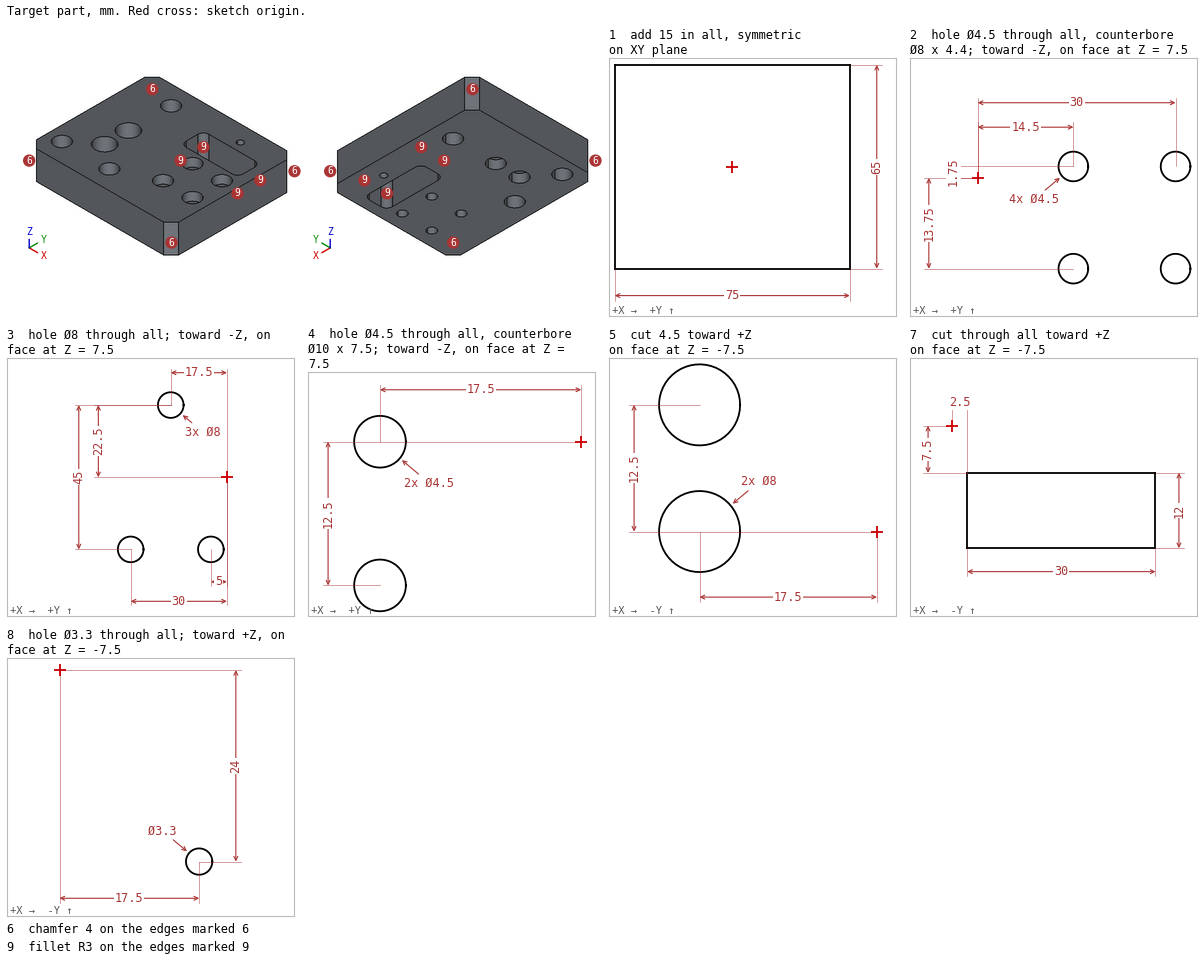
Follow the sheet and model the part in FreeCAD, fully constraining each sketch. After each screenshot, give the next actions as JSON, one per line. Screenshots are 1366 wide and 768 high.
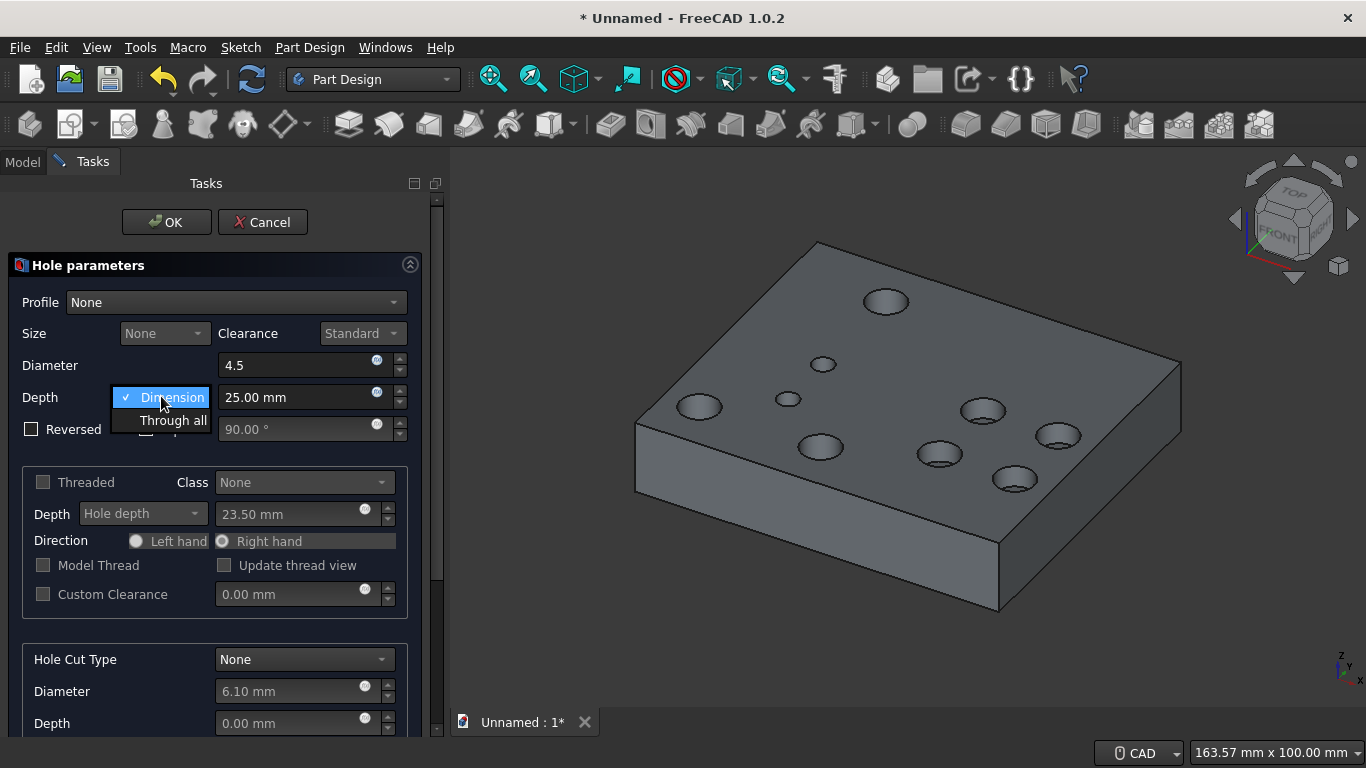
{"action": "left_click", "coordinate": [160, 420]}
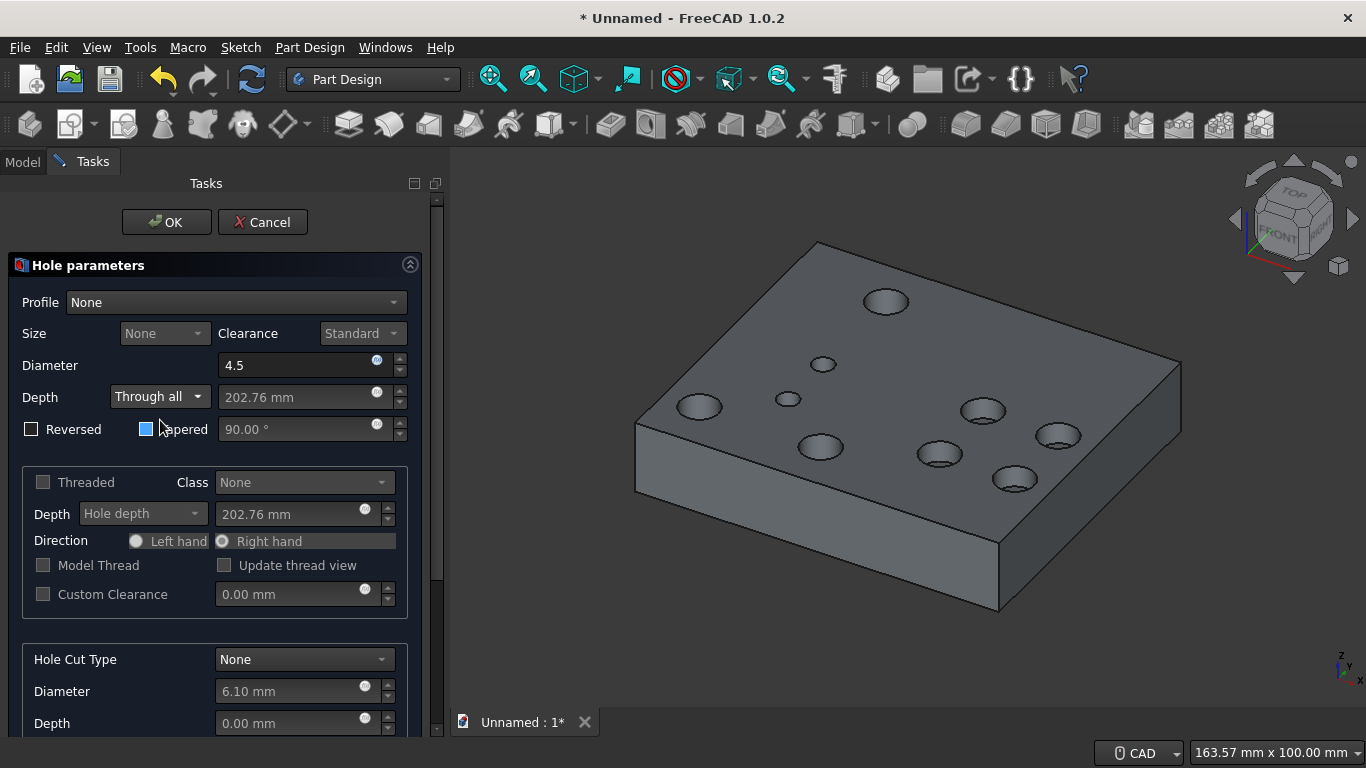
{"action": "left_click", "coordinate": [306, 660]}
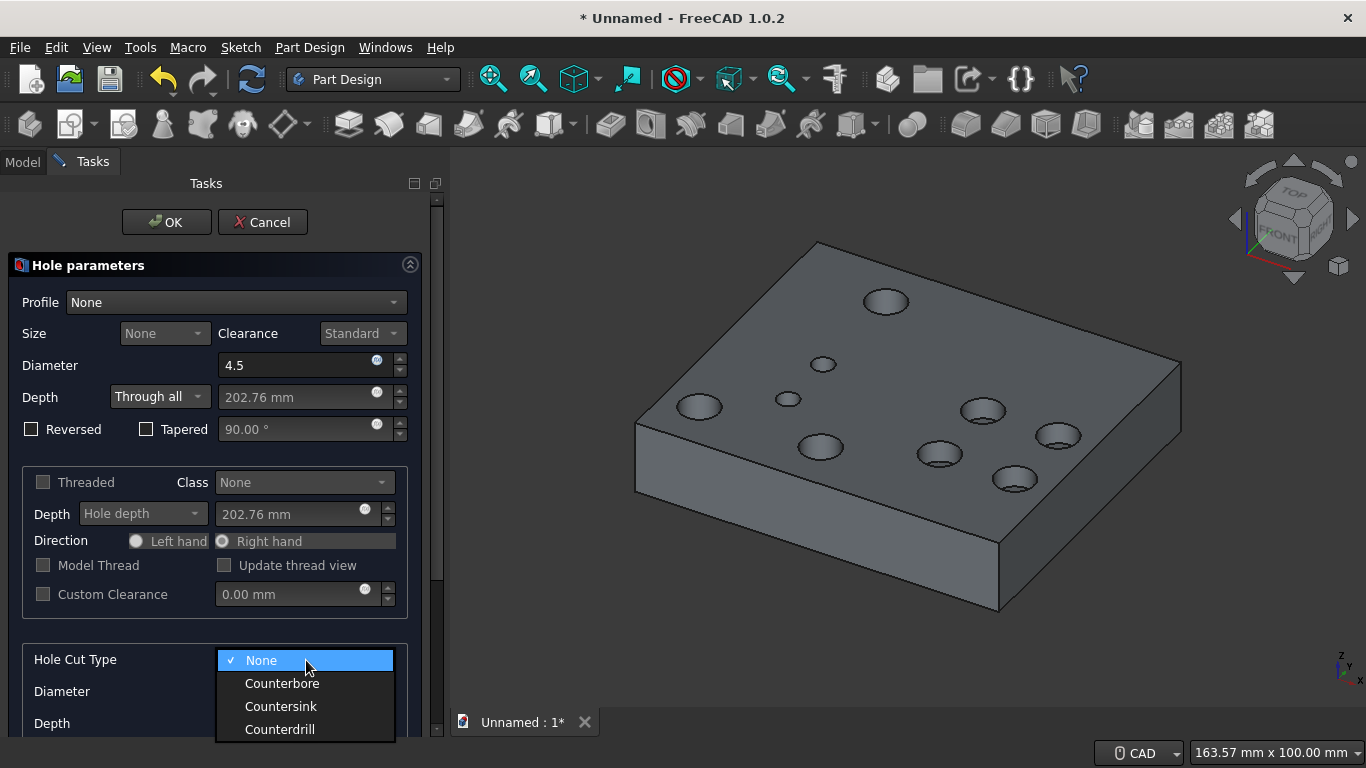
{"action": "left_click", "coordinate": [304, 684]}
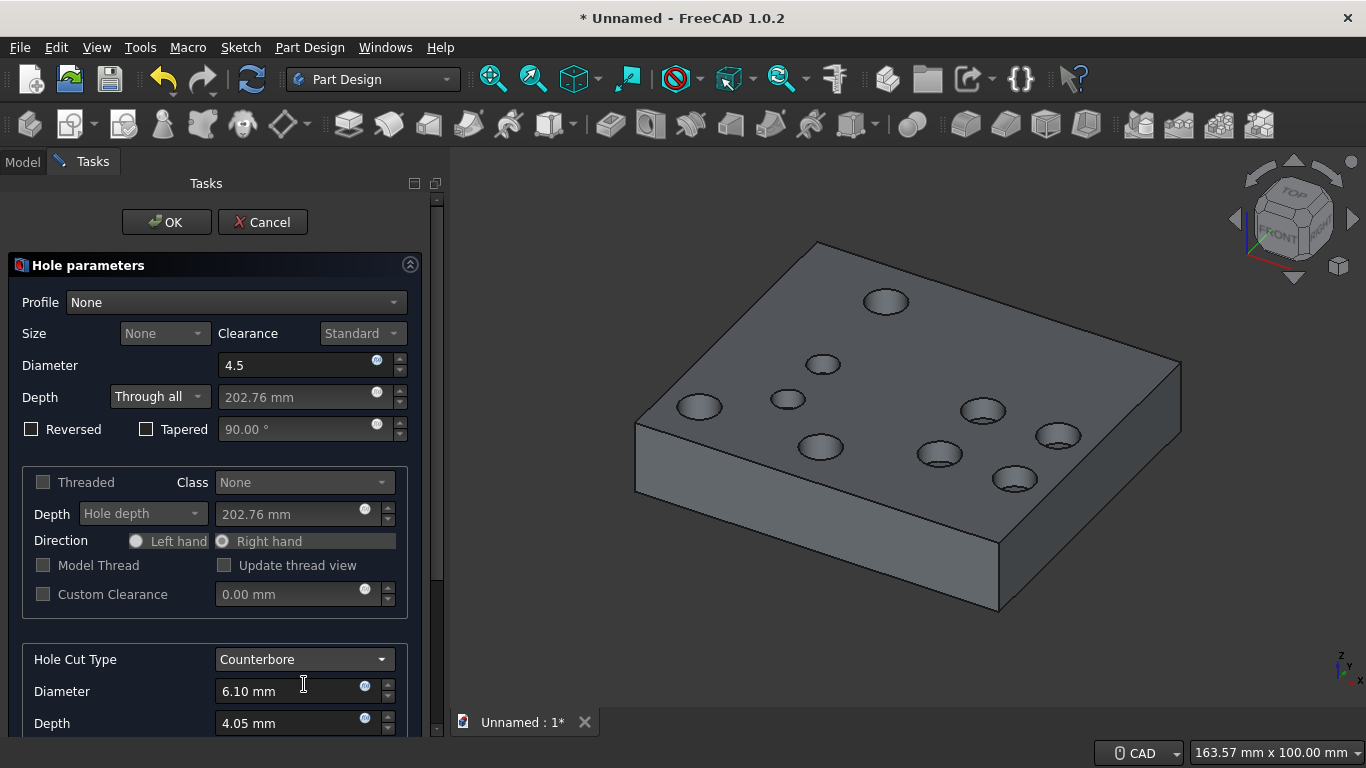
{"action": "triple_click", "coordinate": [298, 691]}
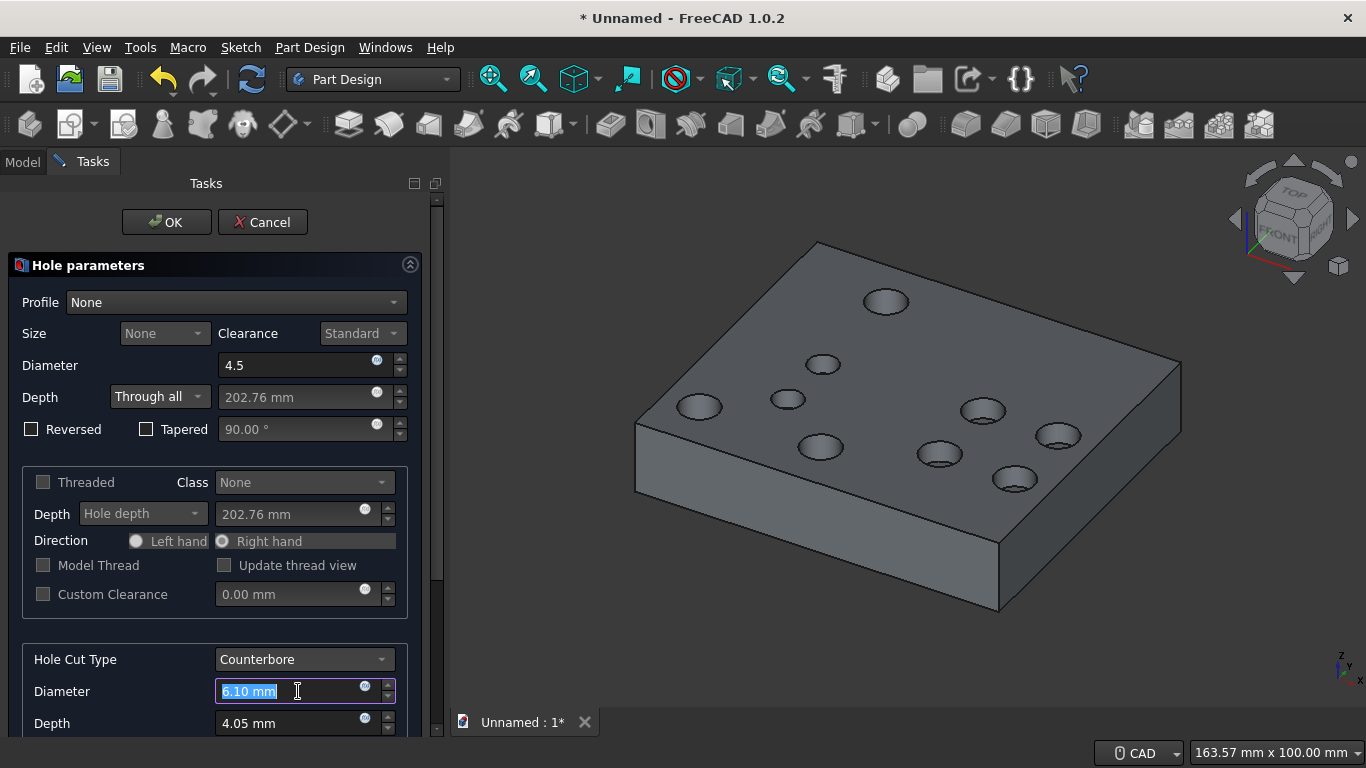
{"action": "type", "text": "10"}
{"action": "key", "text": "Tab"}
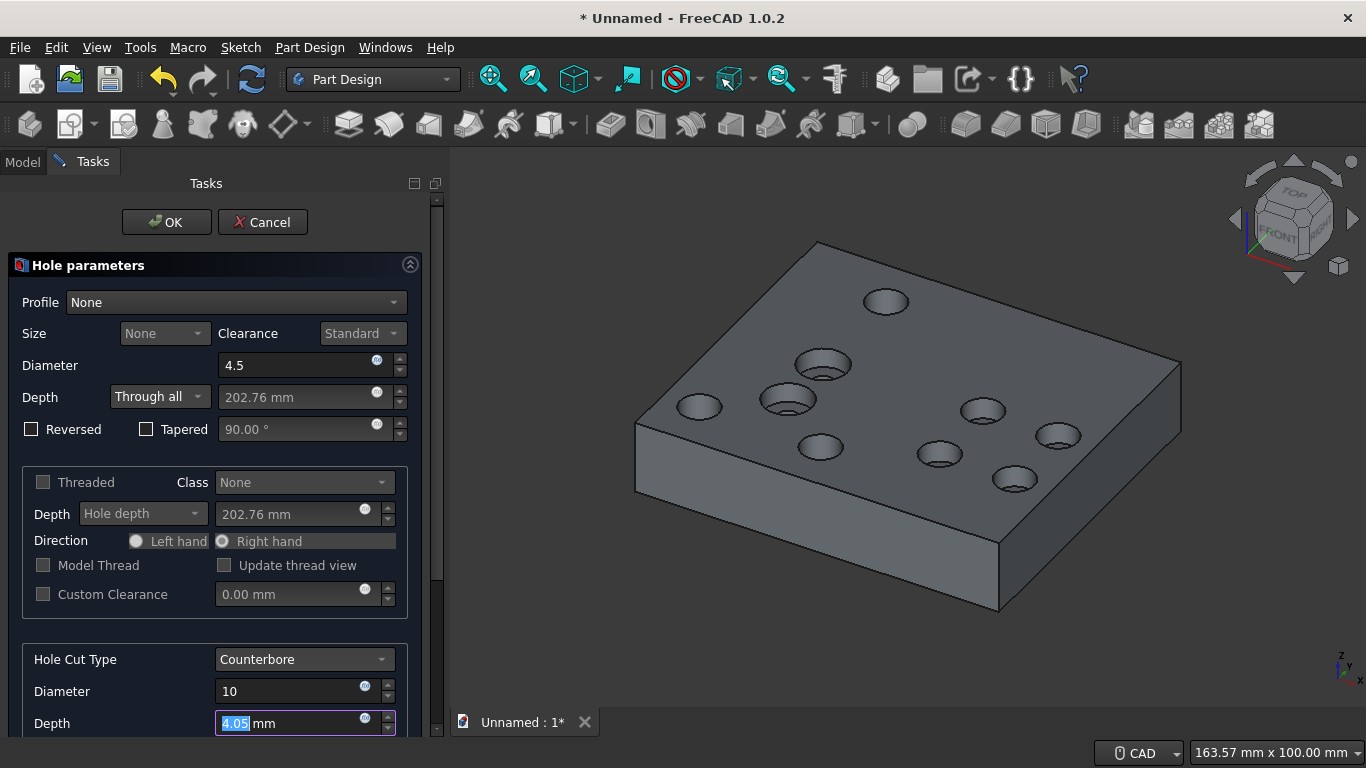
{"action": "type", "text": "7.5"}
{"action": "key", "text": "Tab"}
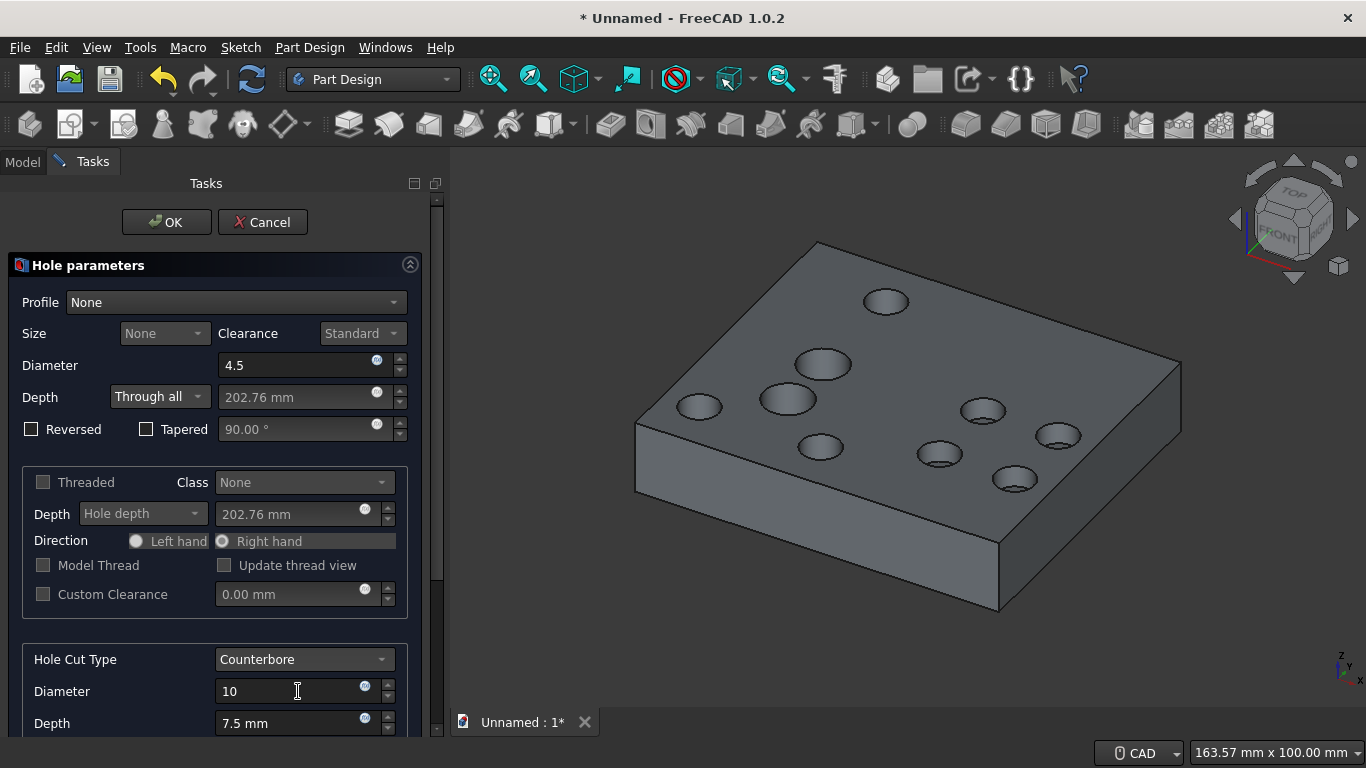
{"action": "left_click", "coordinate": [167, 222]}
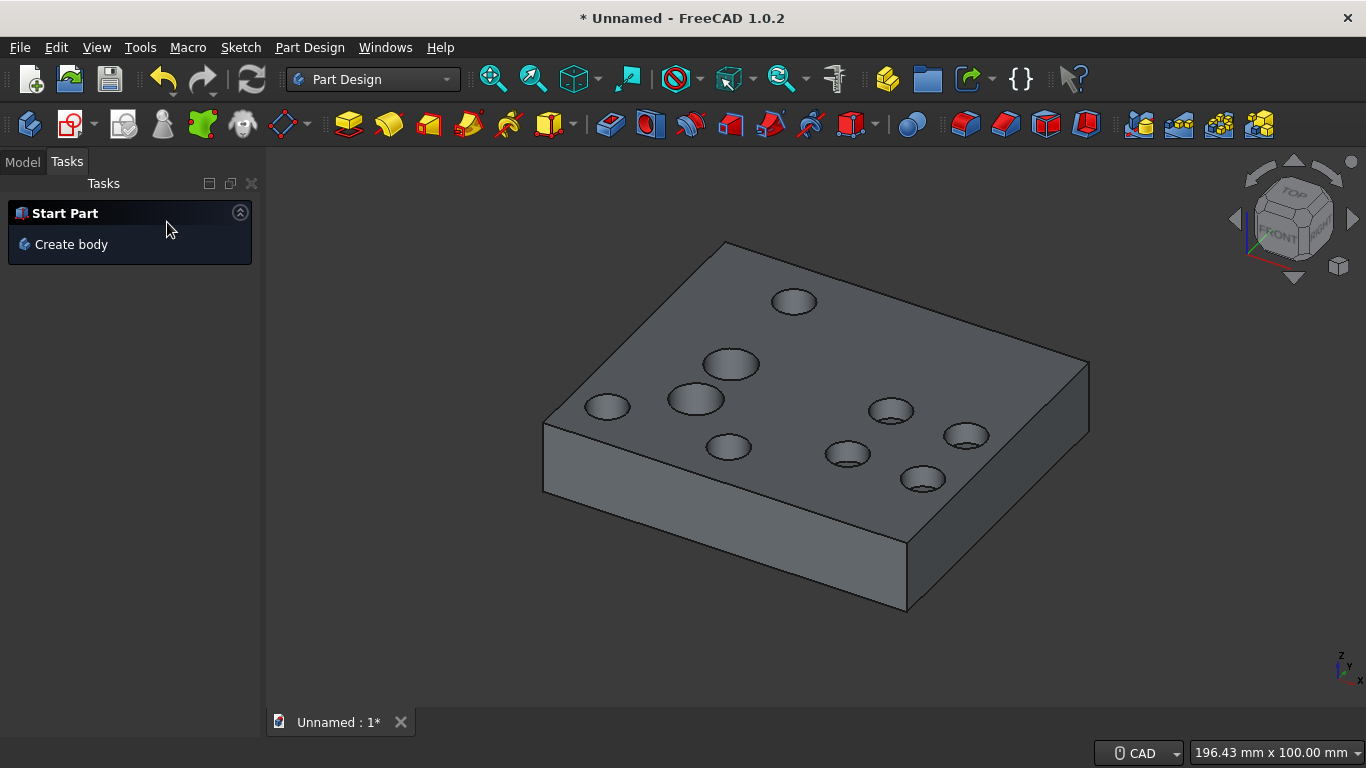
{"action": "key", "text": "5"}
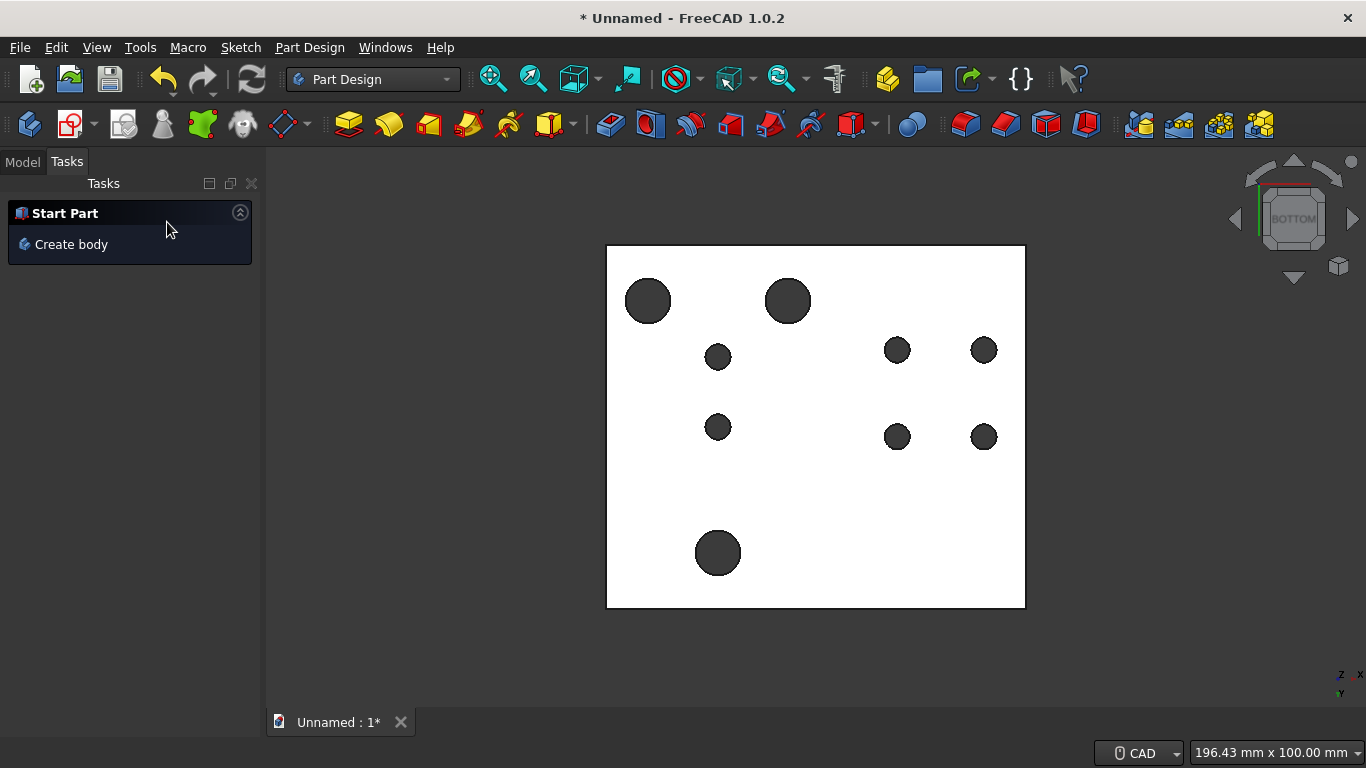
{"action": "left_click", "coordinate": [816, 478]}